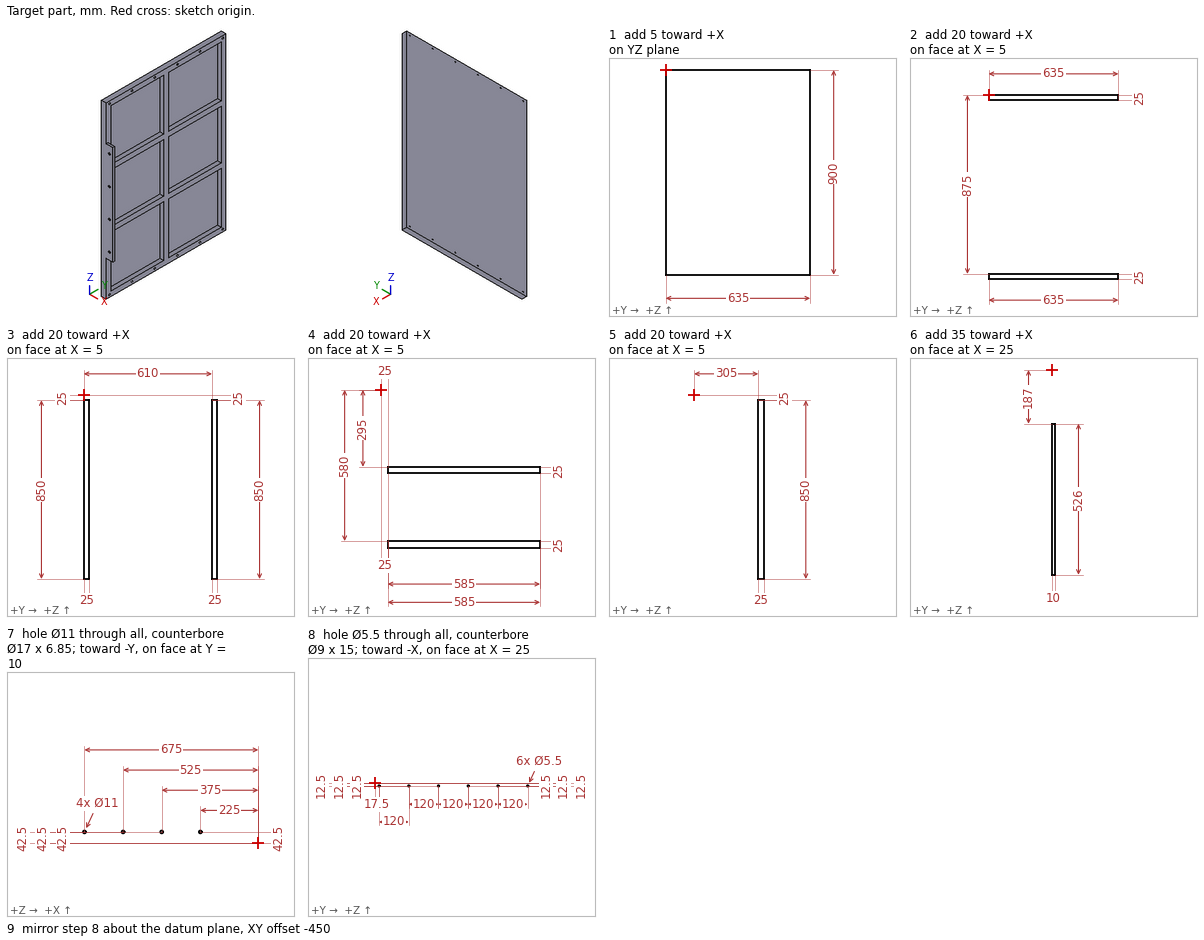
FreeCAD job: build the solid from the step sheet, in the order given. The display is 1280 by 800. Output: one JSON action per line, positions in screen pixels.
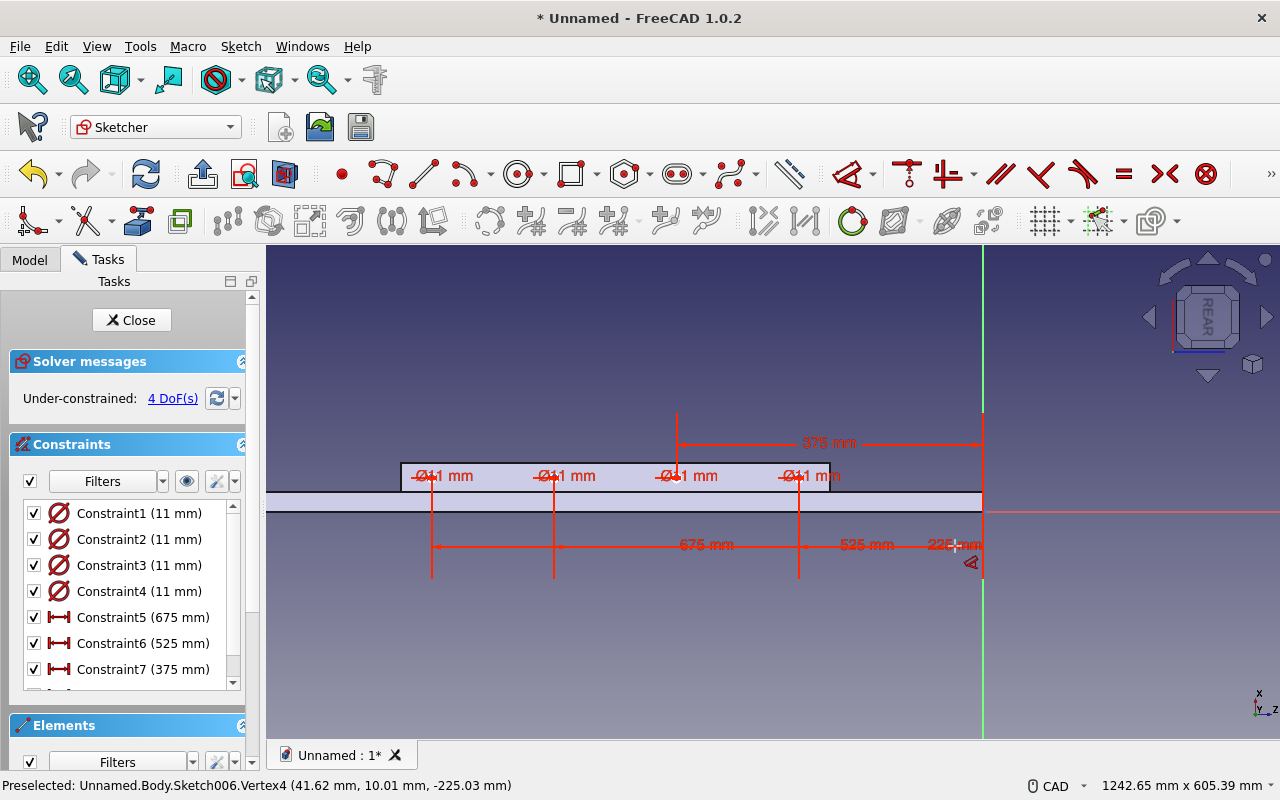
{"action": "left_click", "coordinate": [432, 478]}
{"action": "left_click", "coordinate": [1017, 495]}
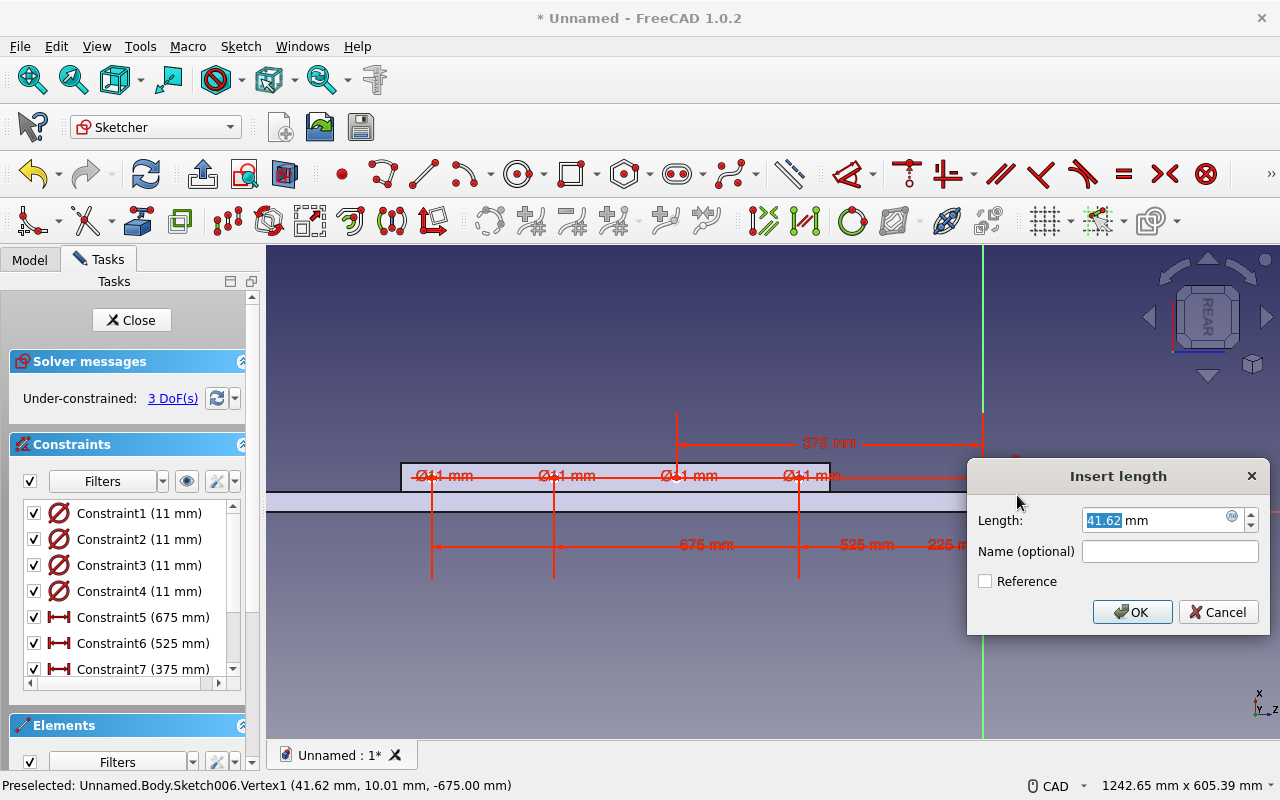
{"action": "type", "text": "42.5"}
{"action": "key", "text": "Return"}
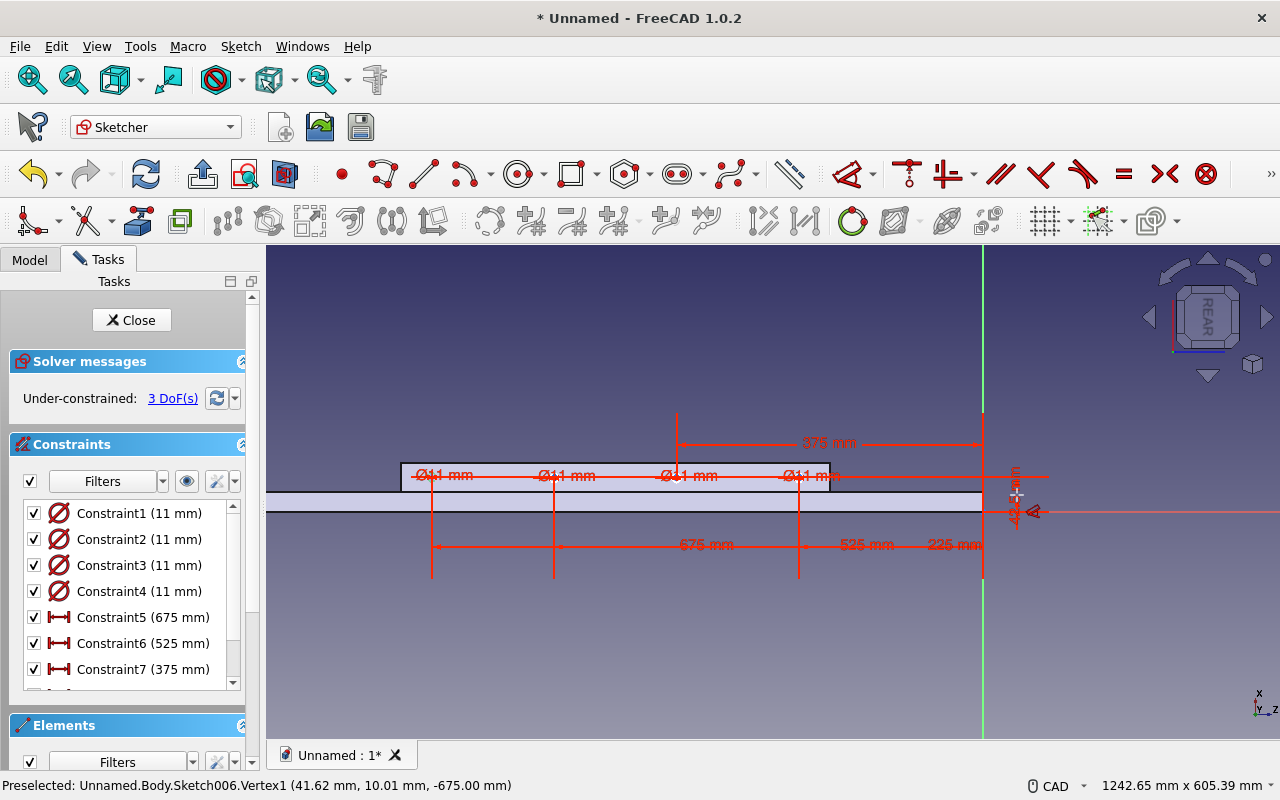
{"action": "left_click", "coordinate": [554, 478]}
{"action": "left_click", "coordinate": [520, 495]}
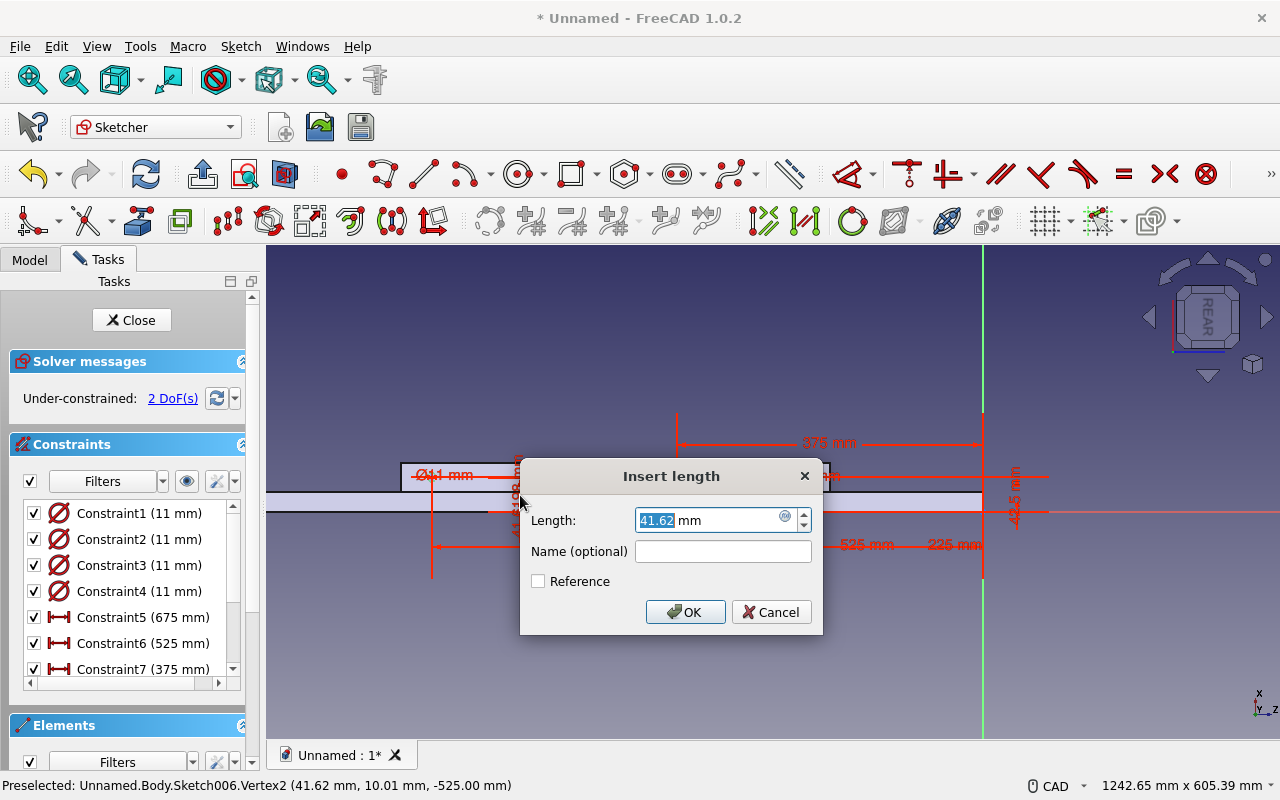
{"action": "type", "text": "42.5"}
{"action": "key", "text": "Return"}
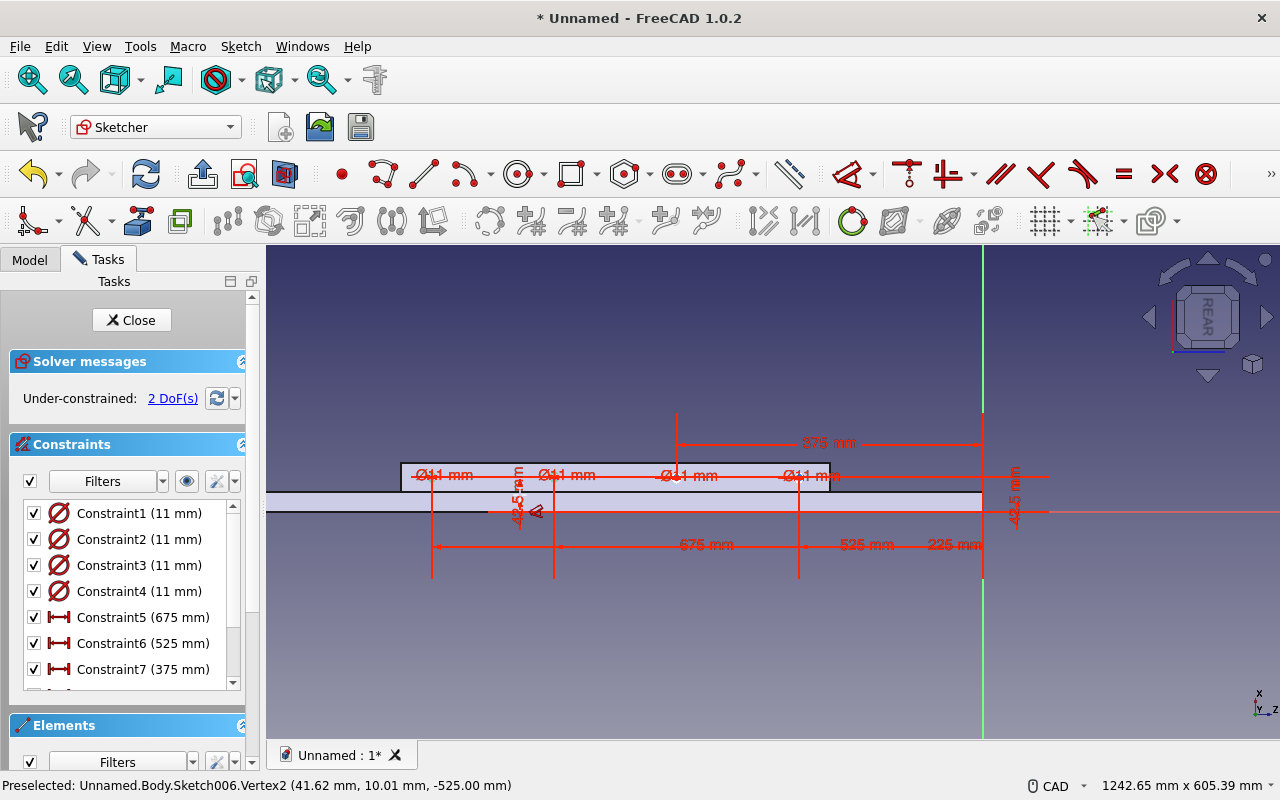
{"action": "left_click", "coordinate": [677, 478]}
{"action": "left_click", "coordinate": [643, 495]}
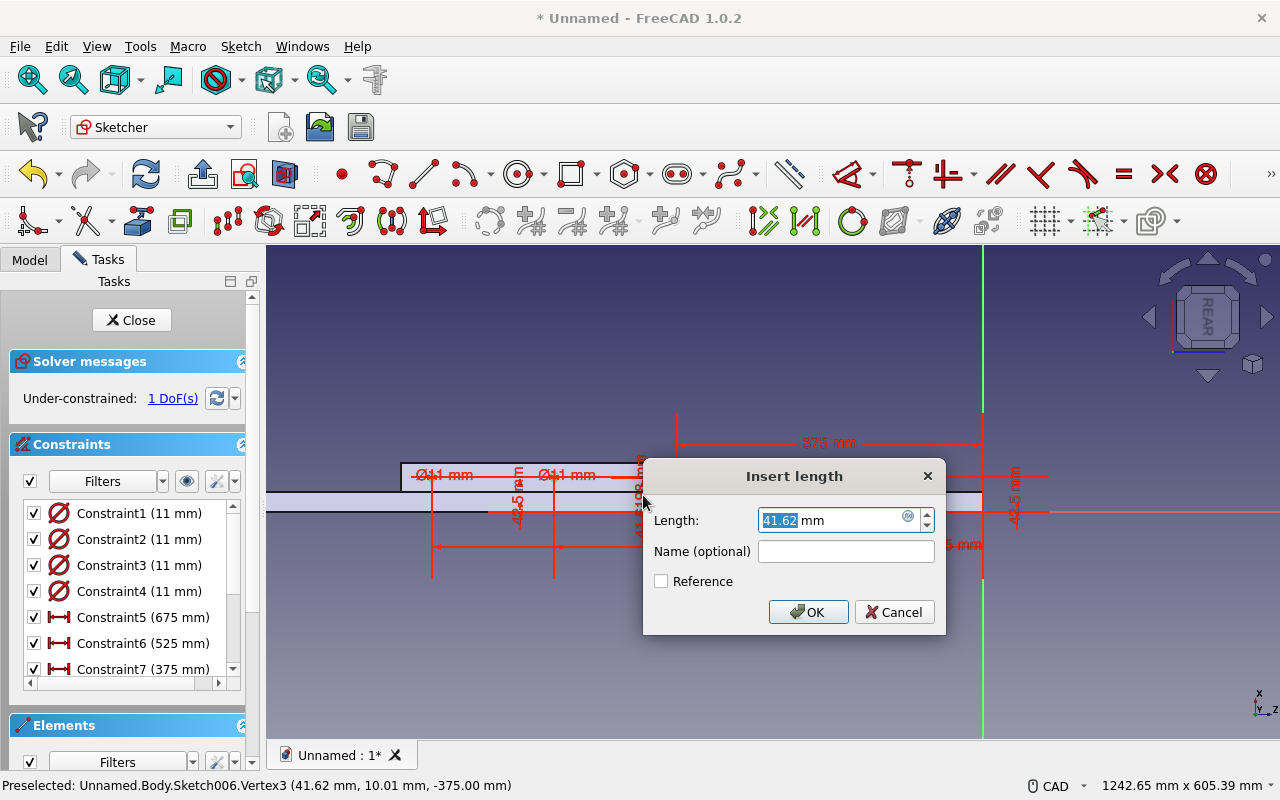
{"action": "type", "text": "42.5"}
{"action": "key", "text": "Return"}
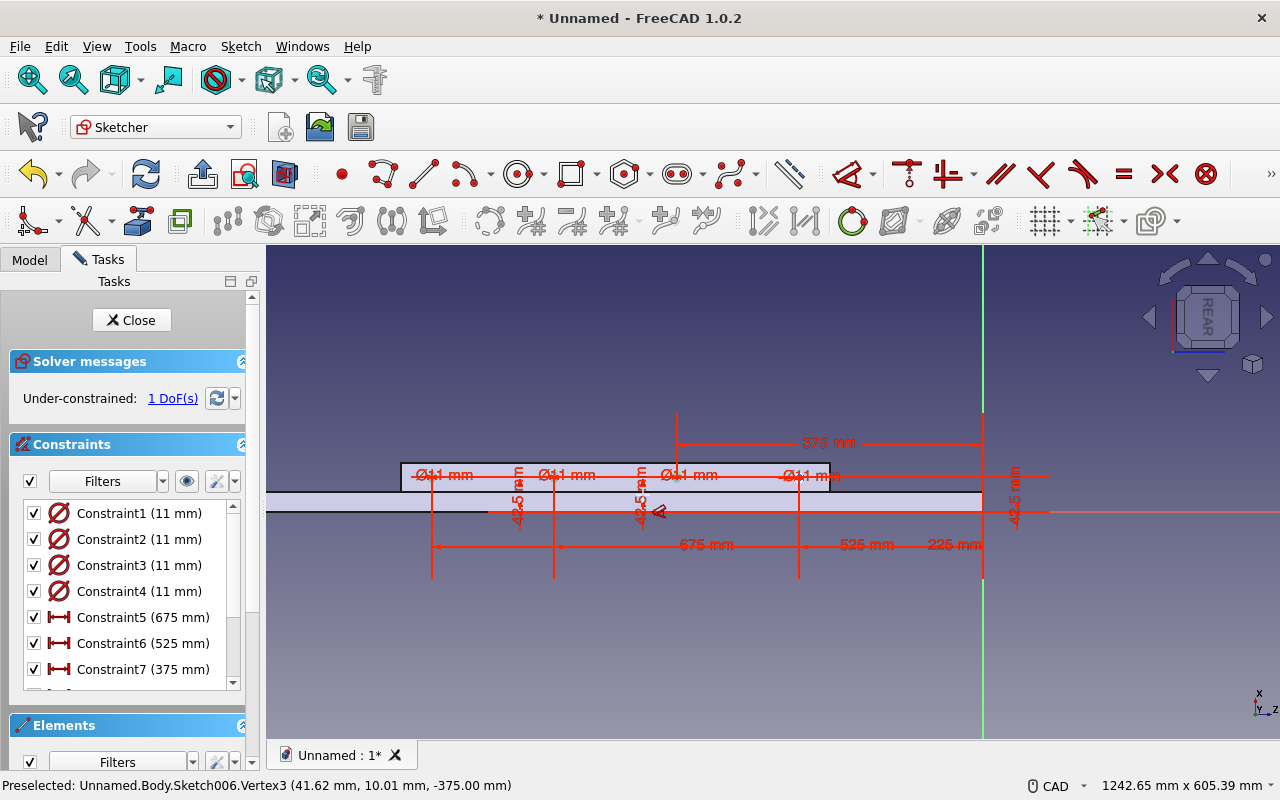
{"action": "left_click", "coordinate": [799, 478]}
{"action": "left_click", "coordinate": [765, 495]}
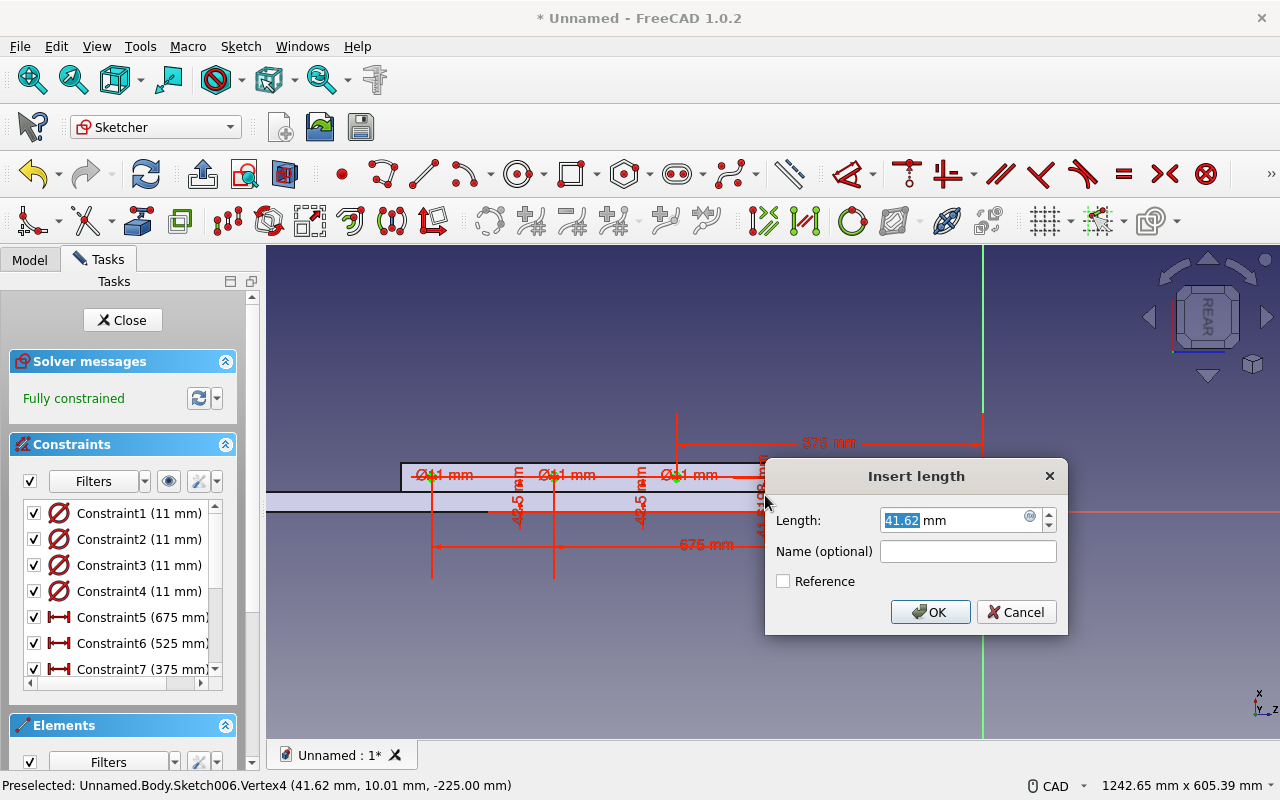
{"action": "type", "text": "42.5"}
{"action": "key", "text": "Return"}
{"action": "key", "text": "Escape"}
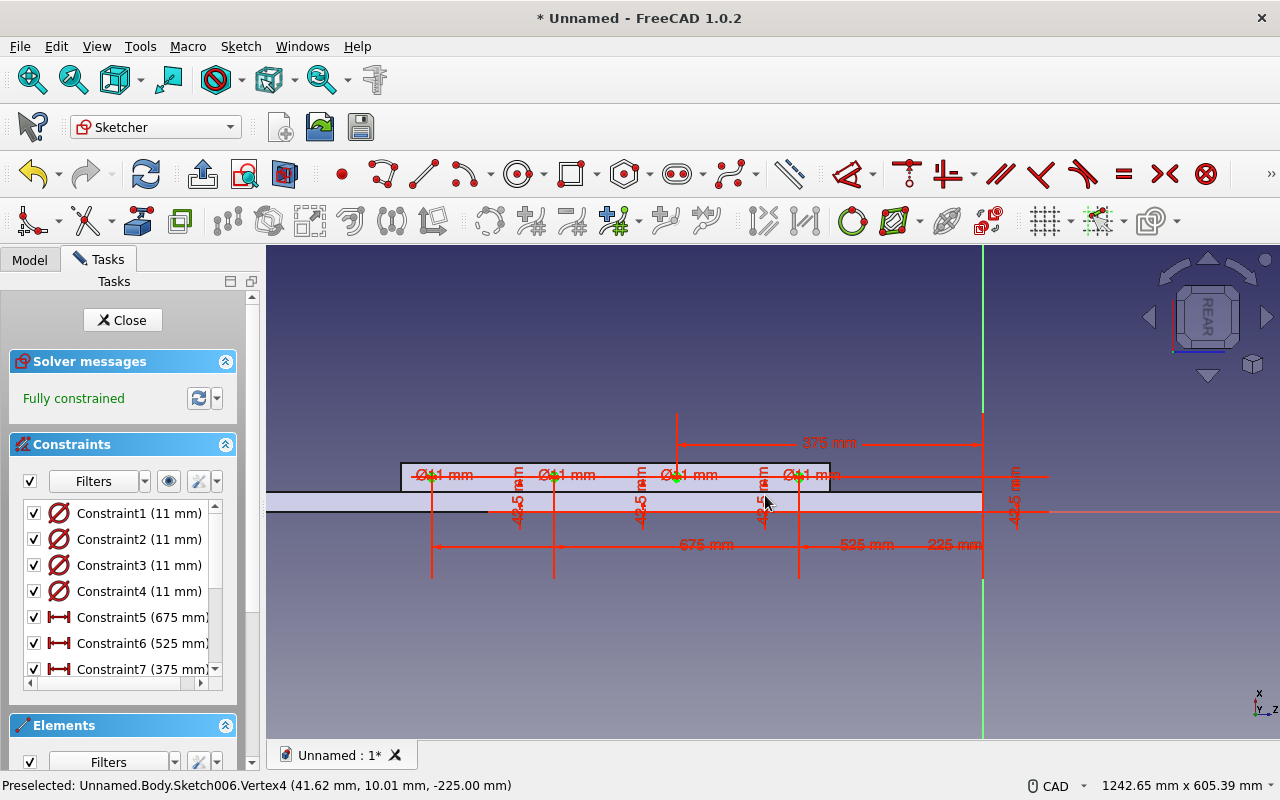
{"action": "left_click", "coordinate": [123, 320]}